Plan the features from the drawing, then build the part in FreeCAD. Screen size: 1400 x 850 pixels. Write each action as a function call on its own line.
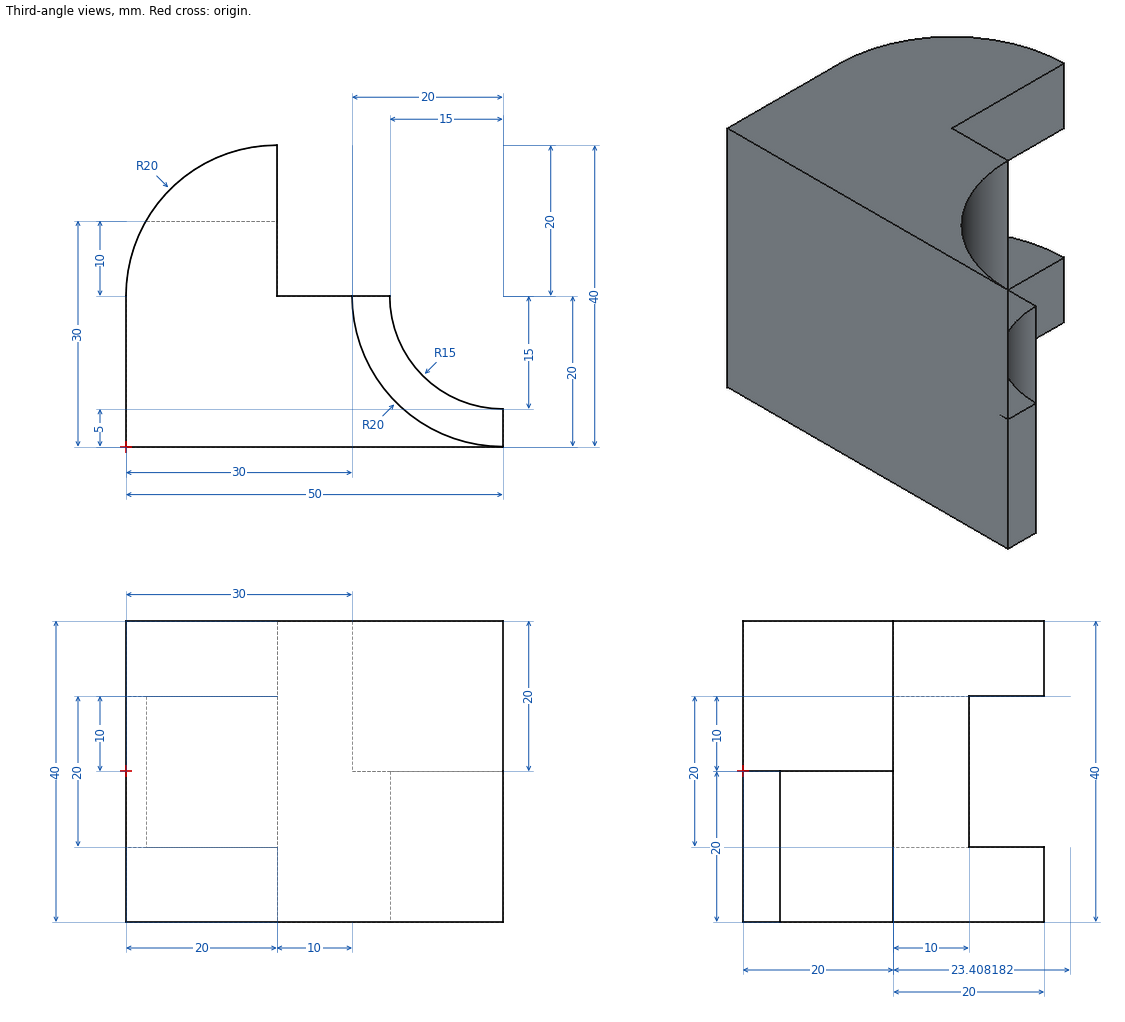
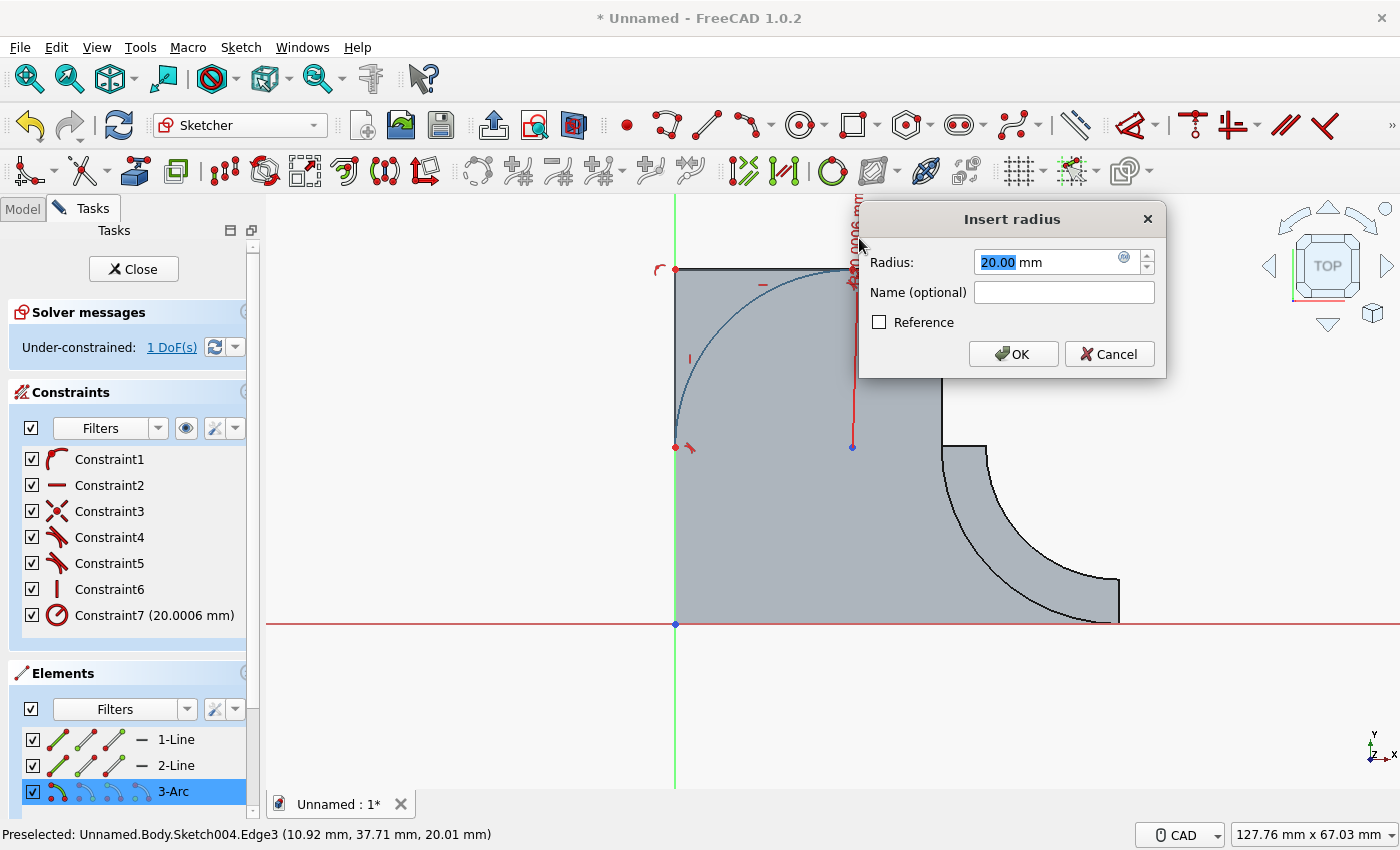
text(20)
key(Return)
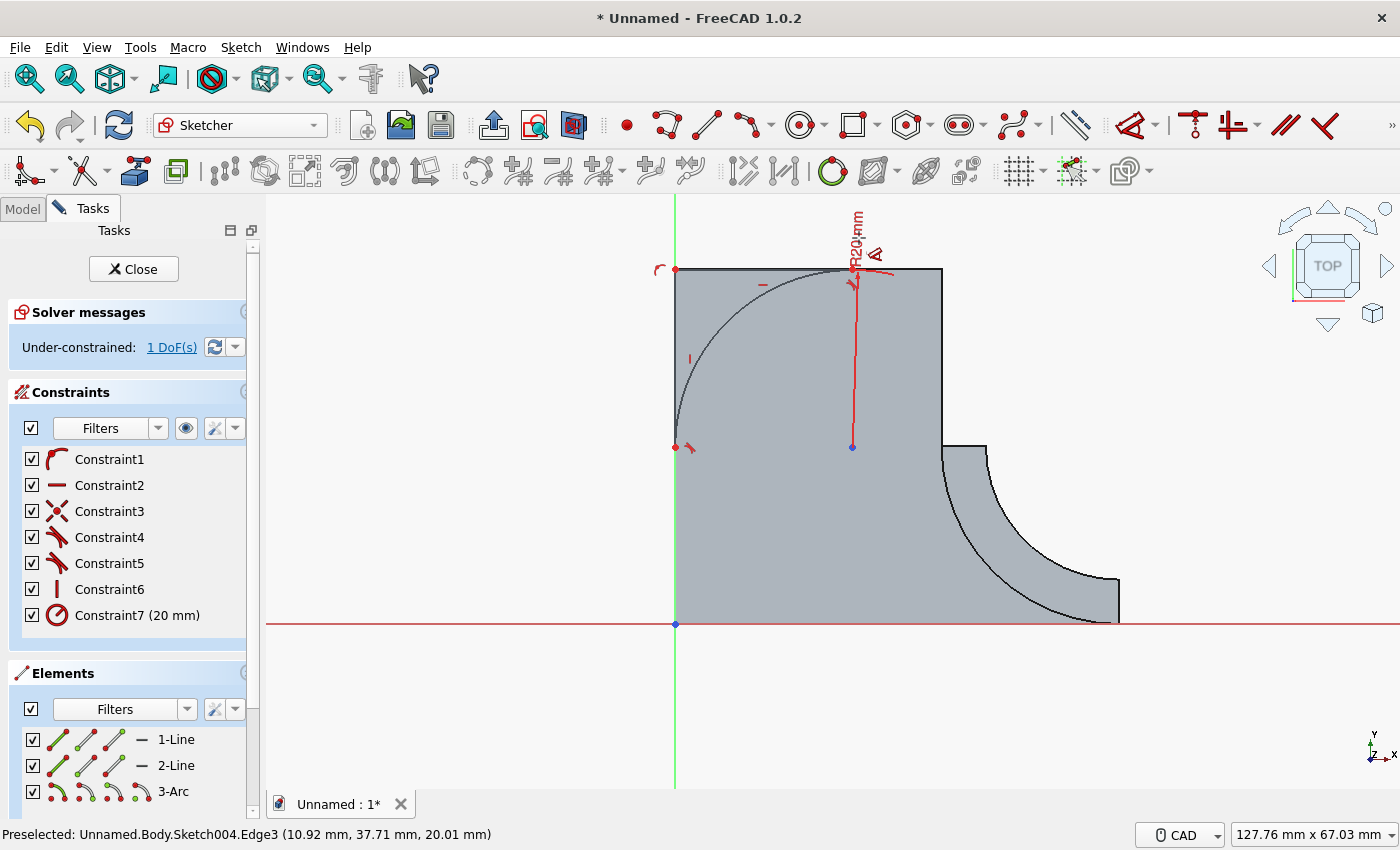
click(853, 270)
click(887, 447)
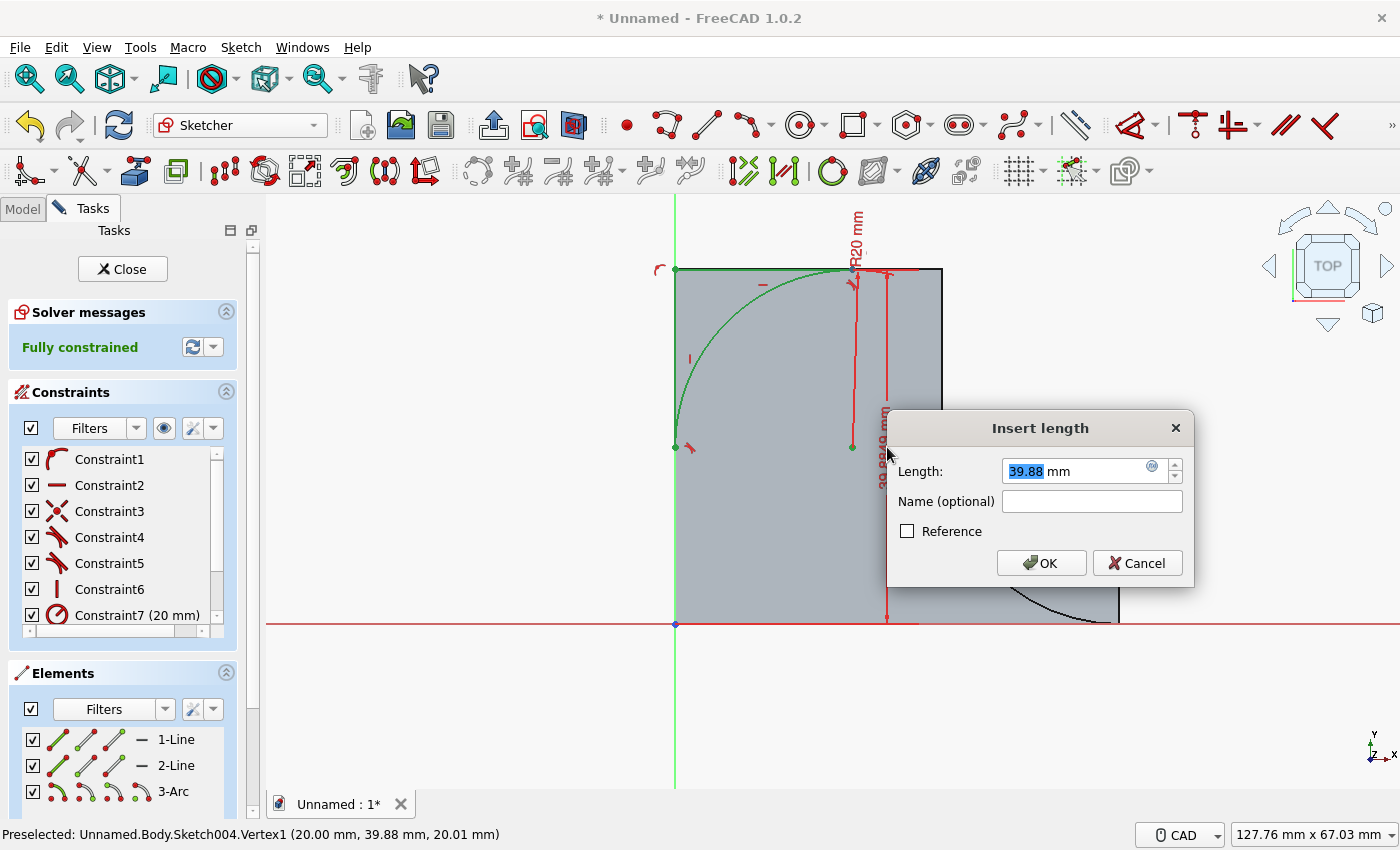
text(40)
key(Return)
key(Escape)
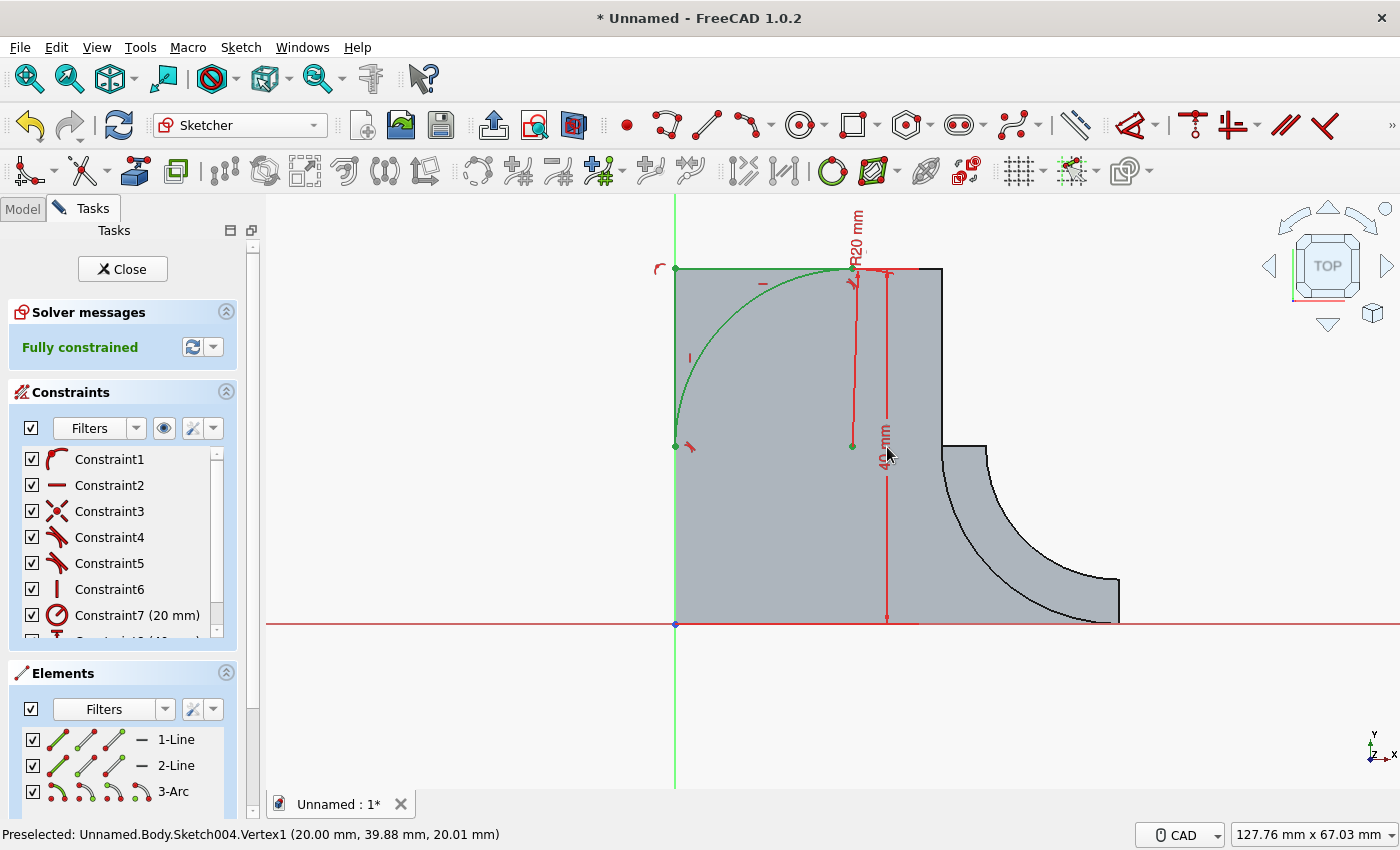
click(123, 269)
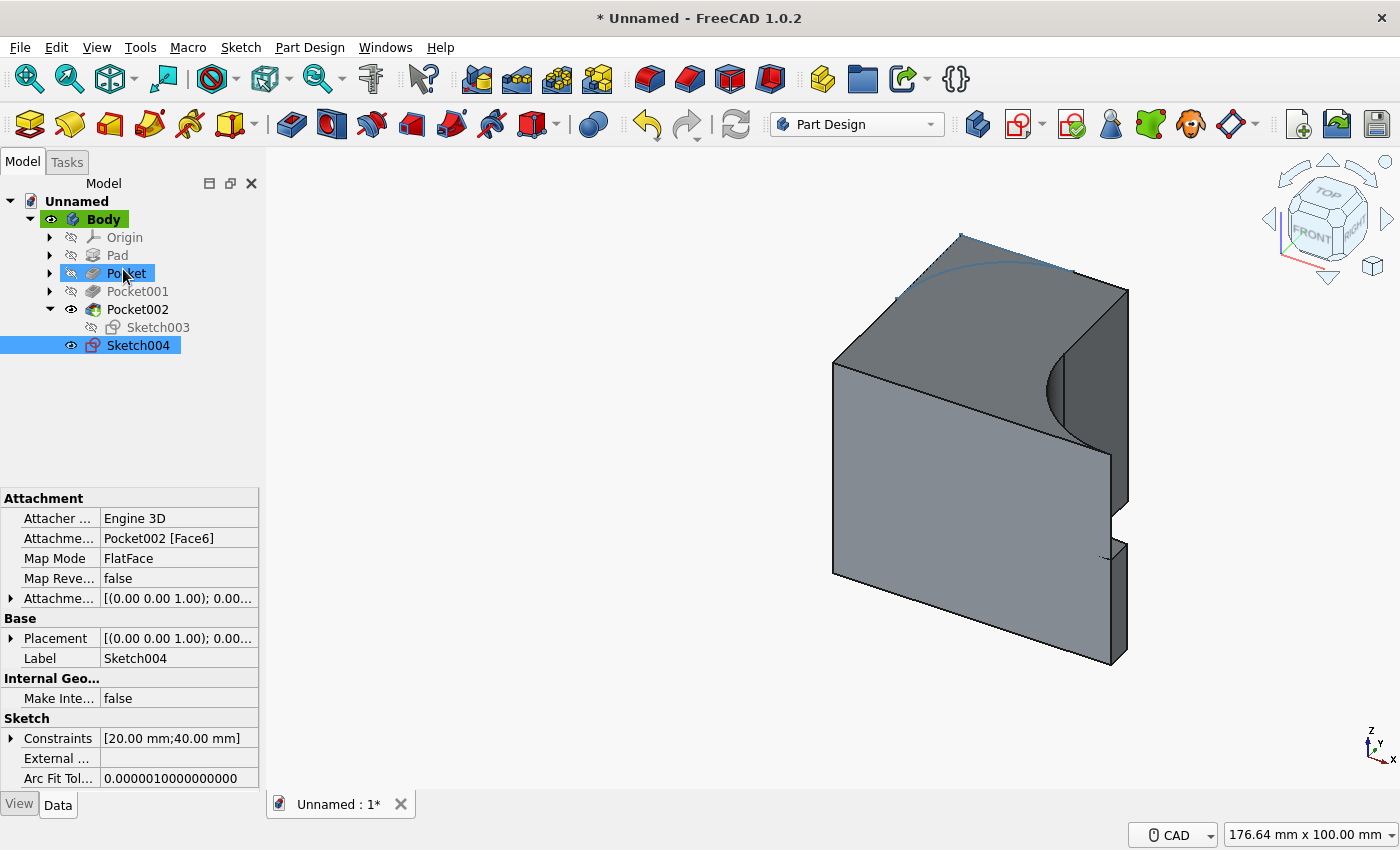
click(292, 124)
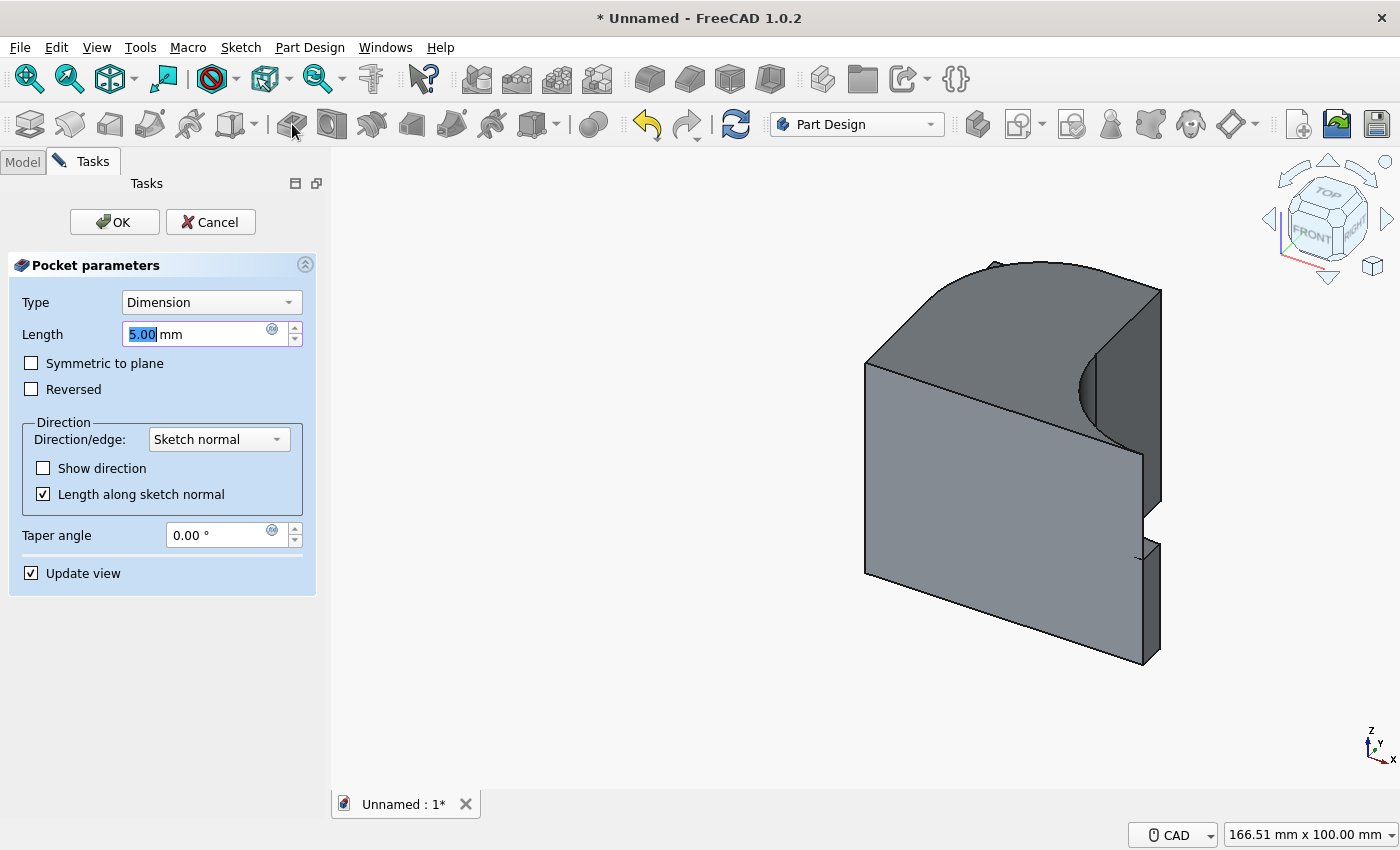
click(212, 302)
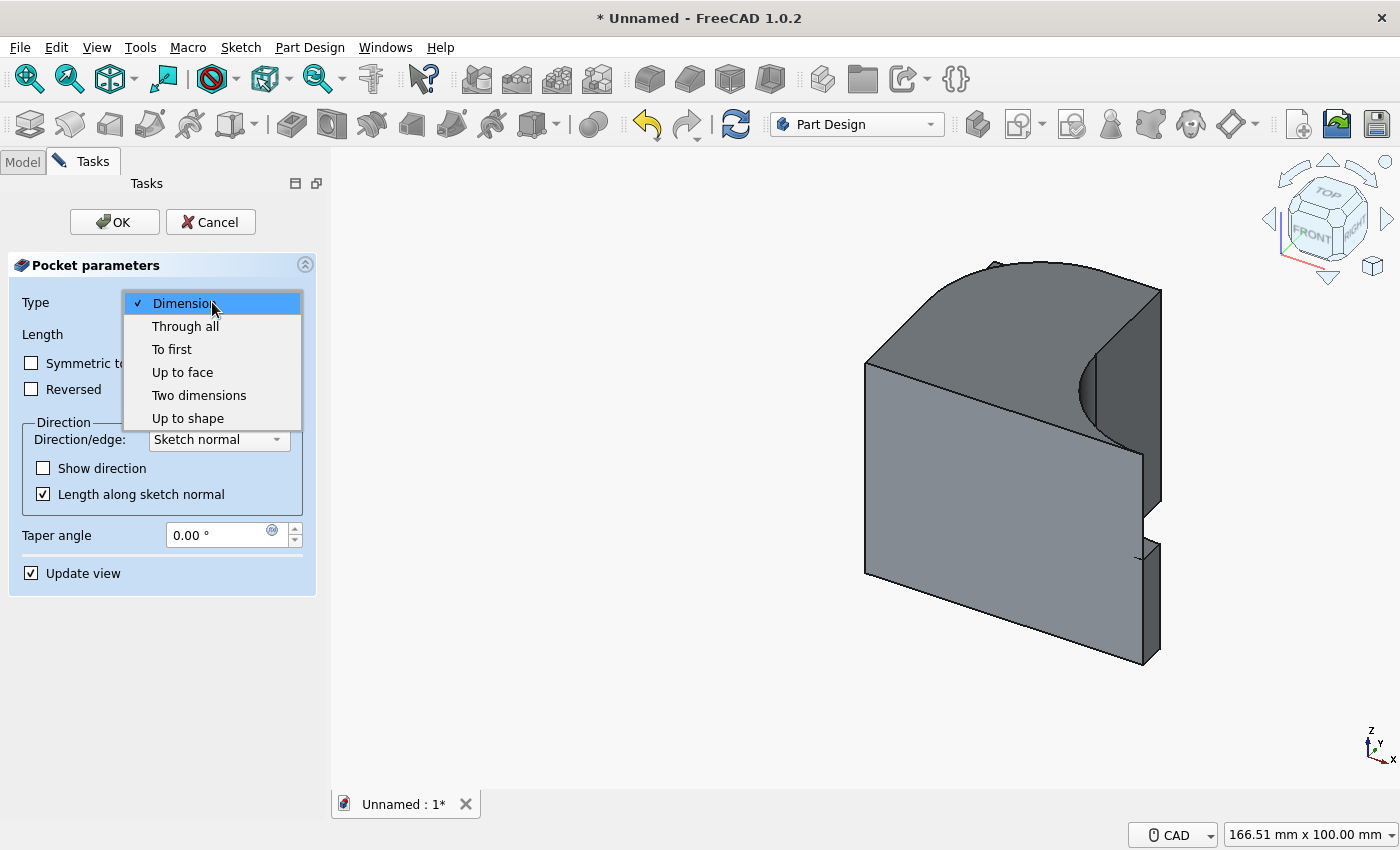
click(212, 326)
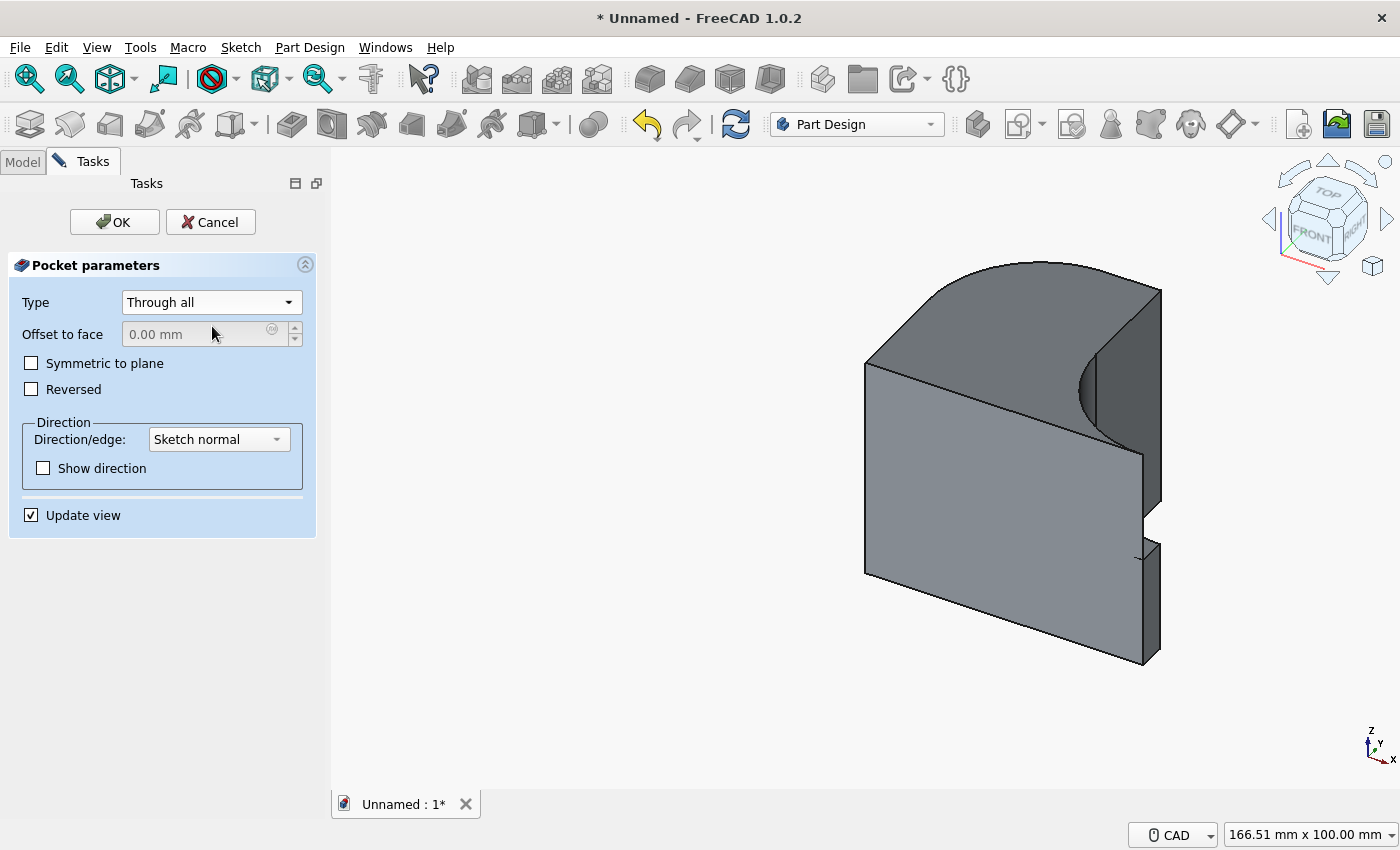
click(115, 222)